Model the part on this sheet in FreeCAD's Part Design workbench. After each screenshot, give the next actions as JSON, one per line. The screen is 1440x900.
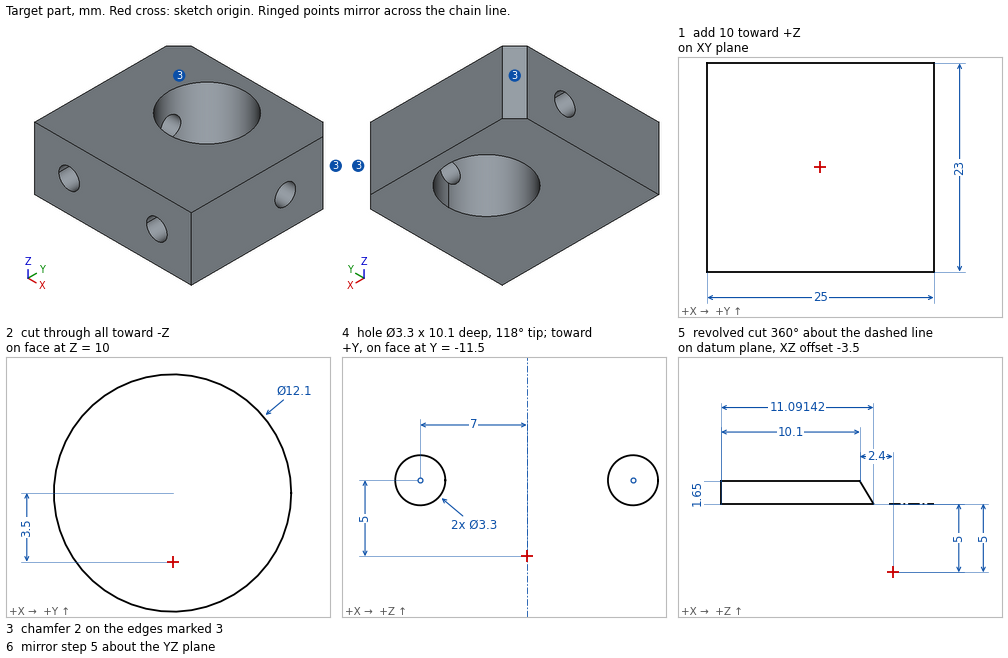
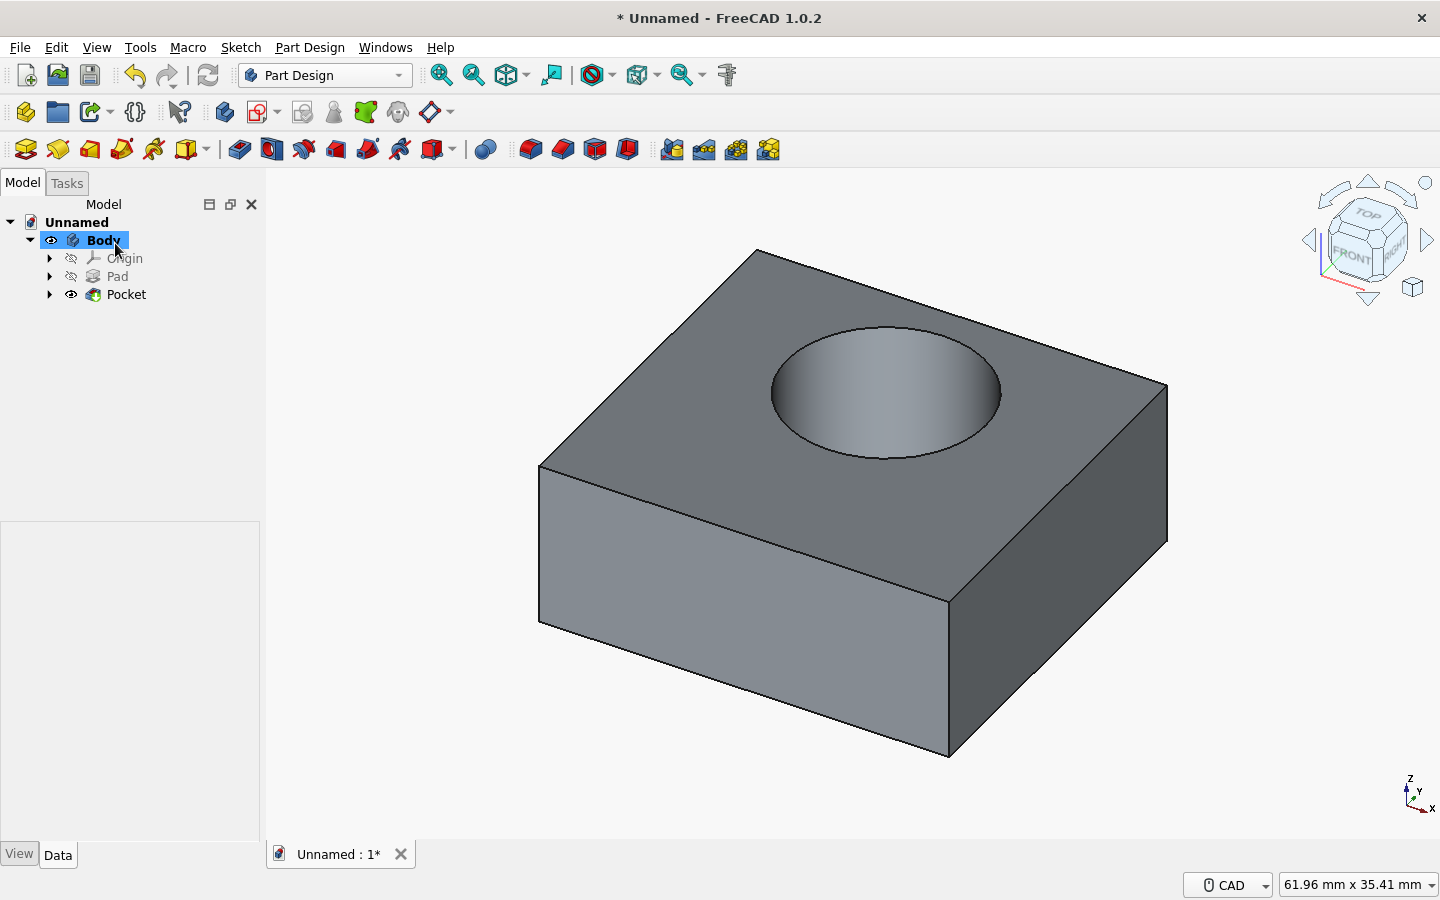
{"action": "key", "text": "0"}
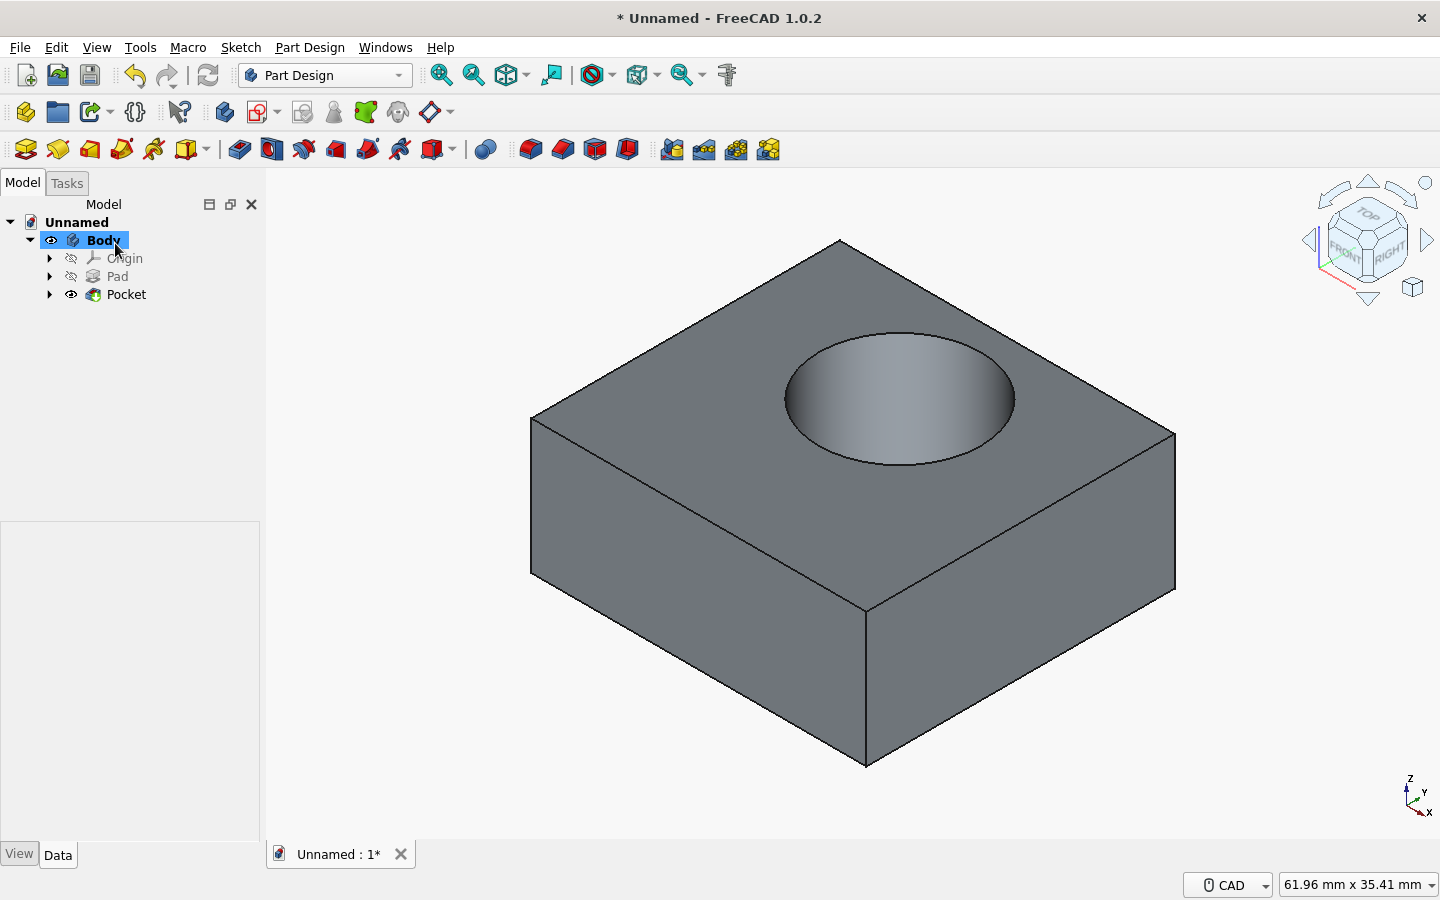
{"action": "key", "text": "2"}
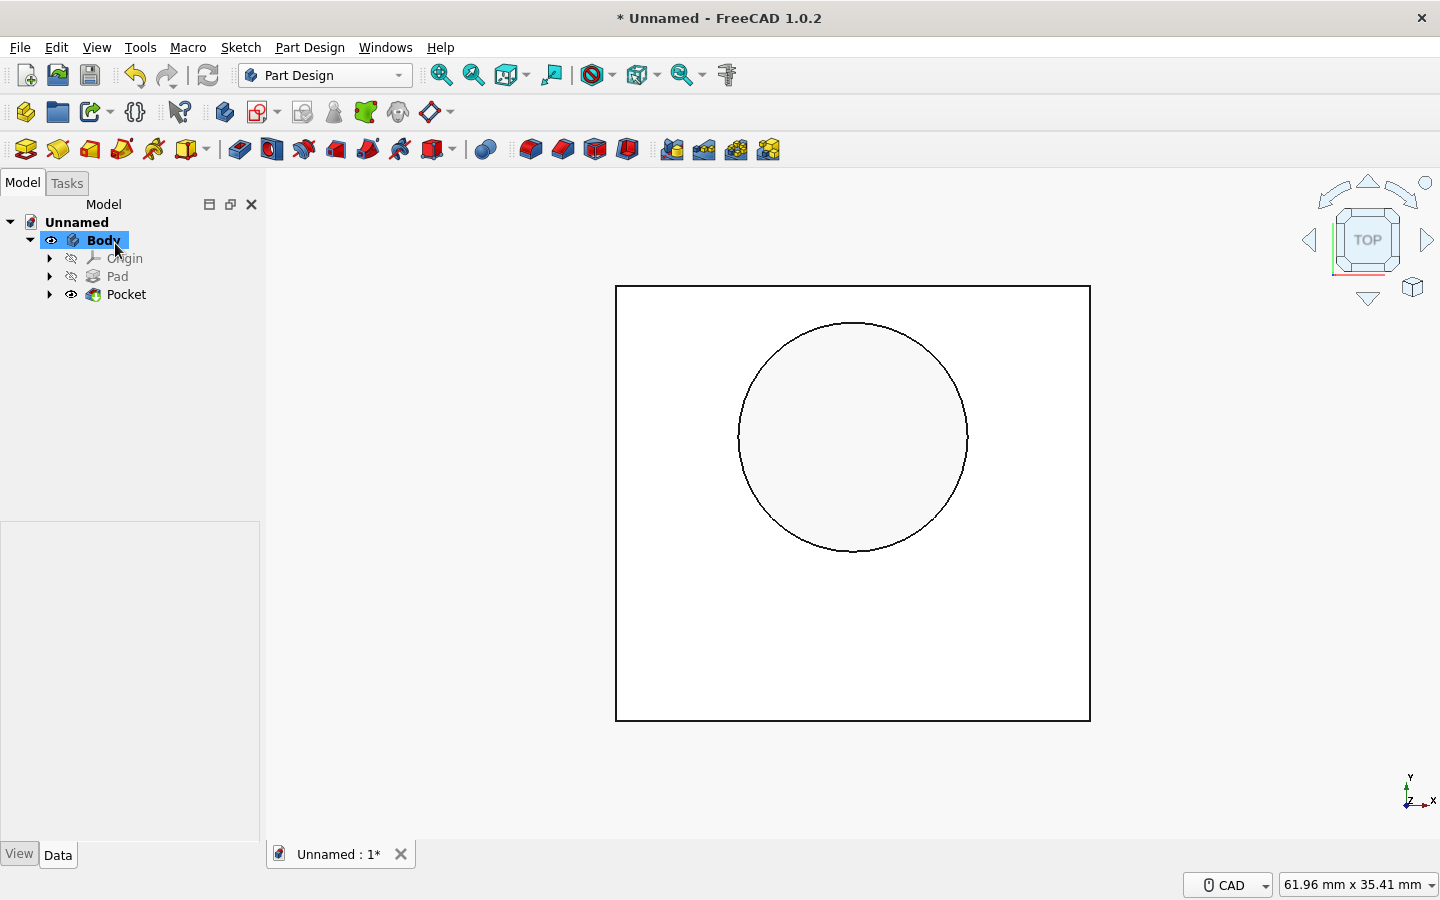
{"action": "key", "text": "1"}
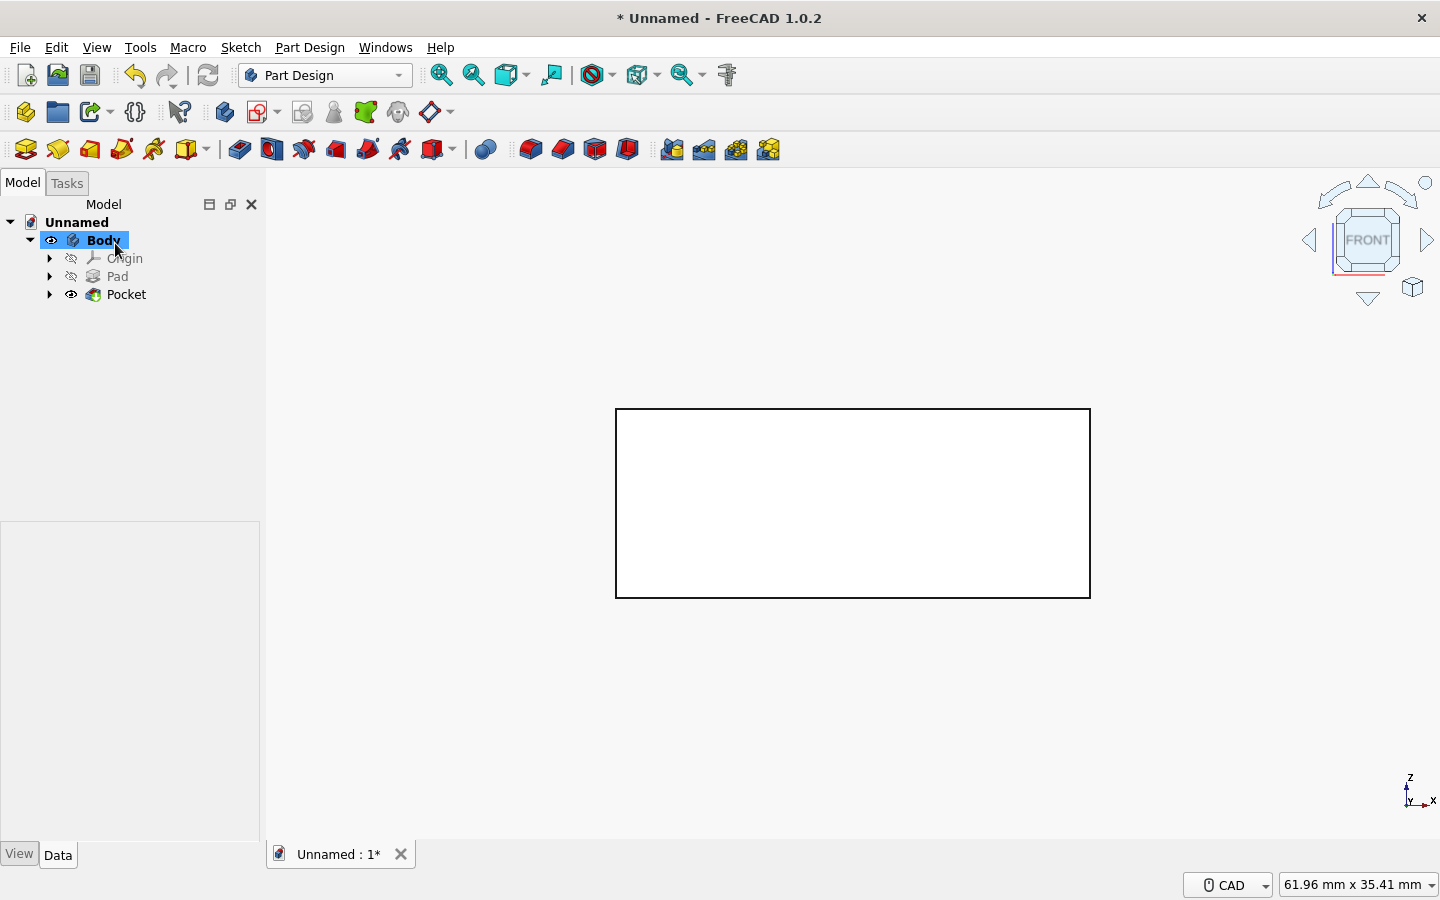
{"action": "left_click", "coordinate": [442, 76]}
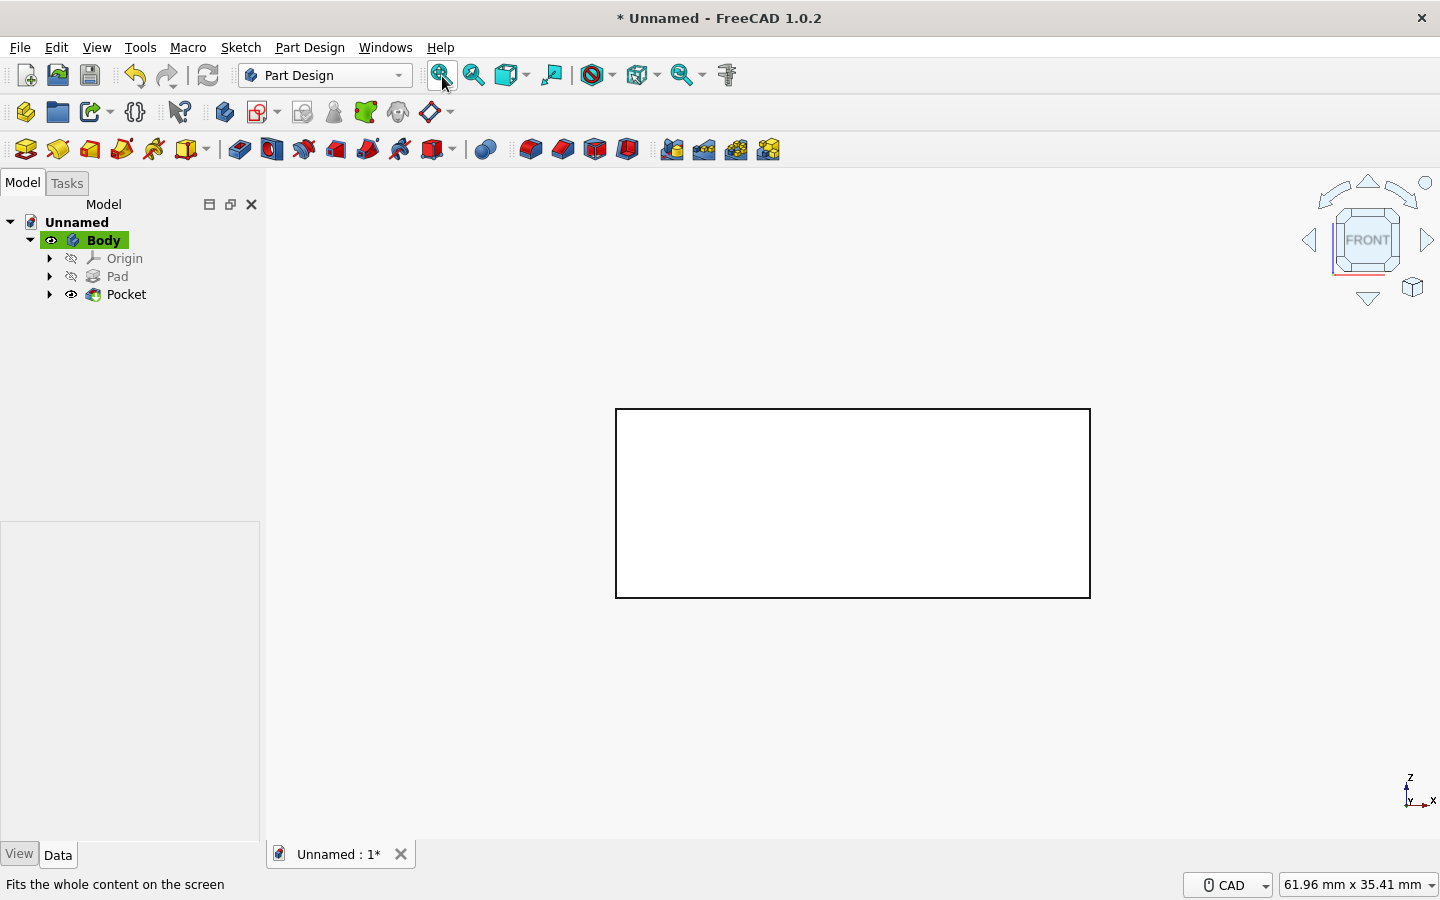
{"action": "key", "text": "3"}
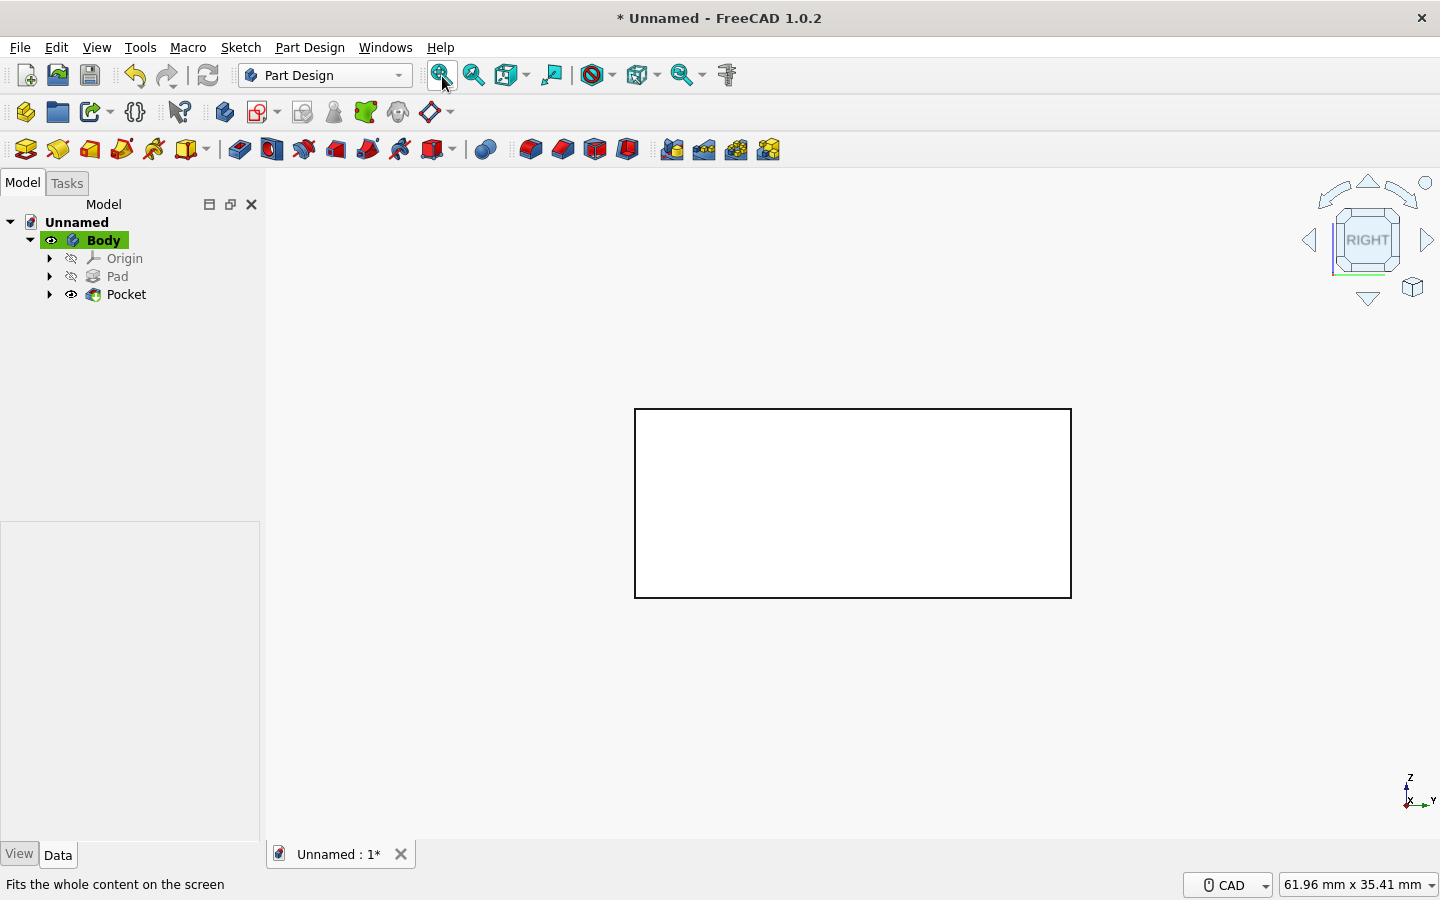
{"action": "key", "text": "v f"}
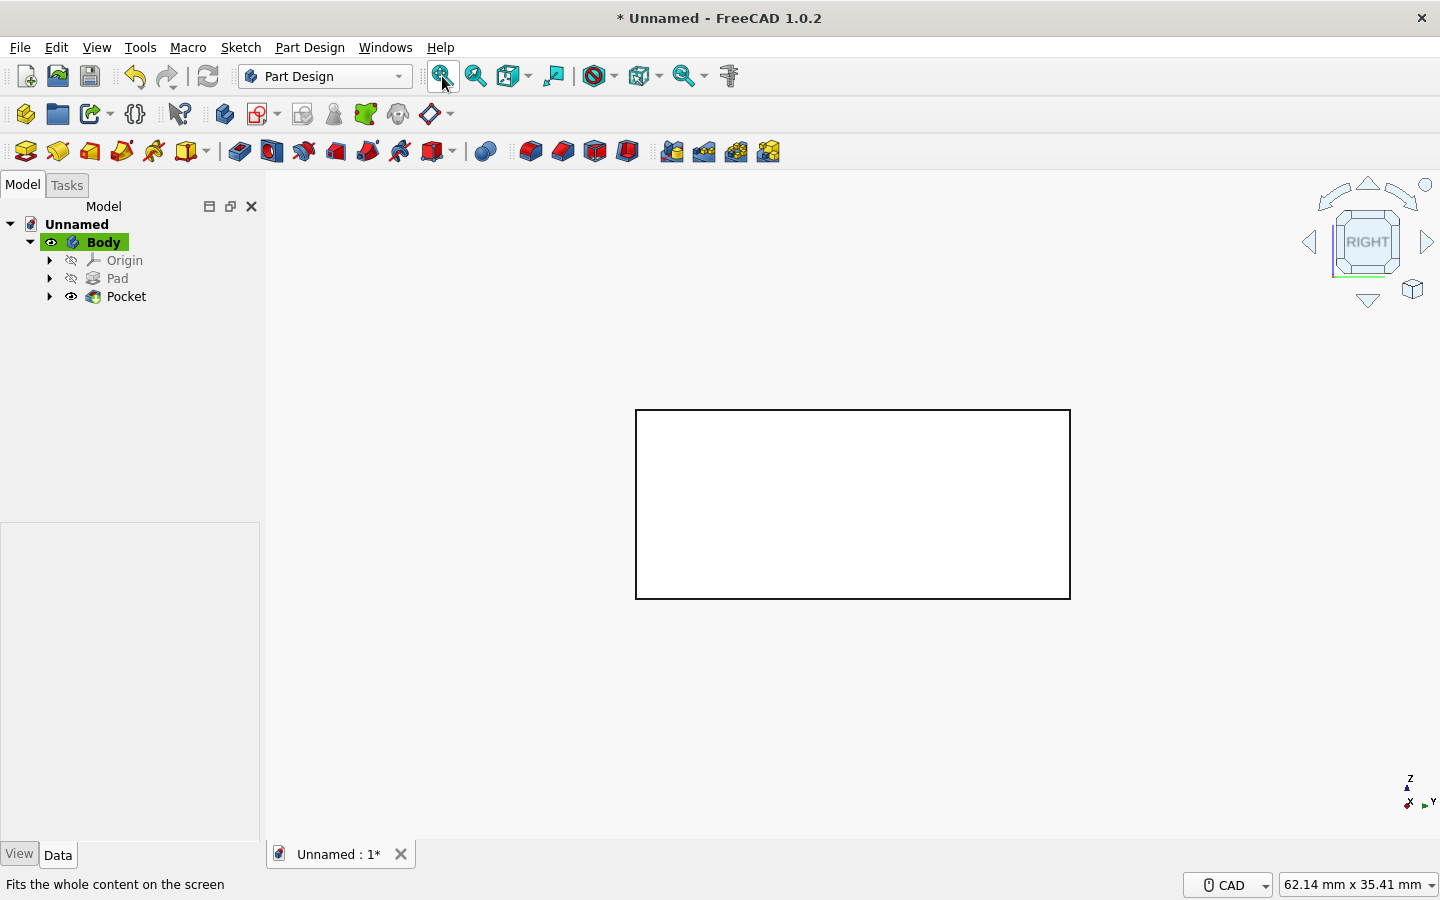
{"action": "left_click", "coordinate": [1070, 503]}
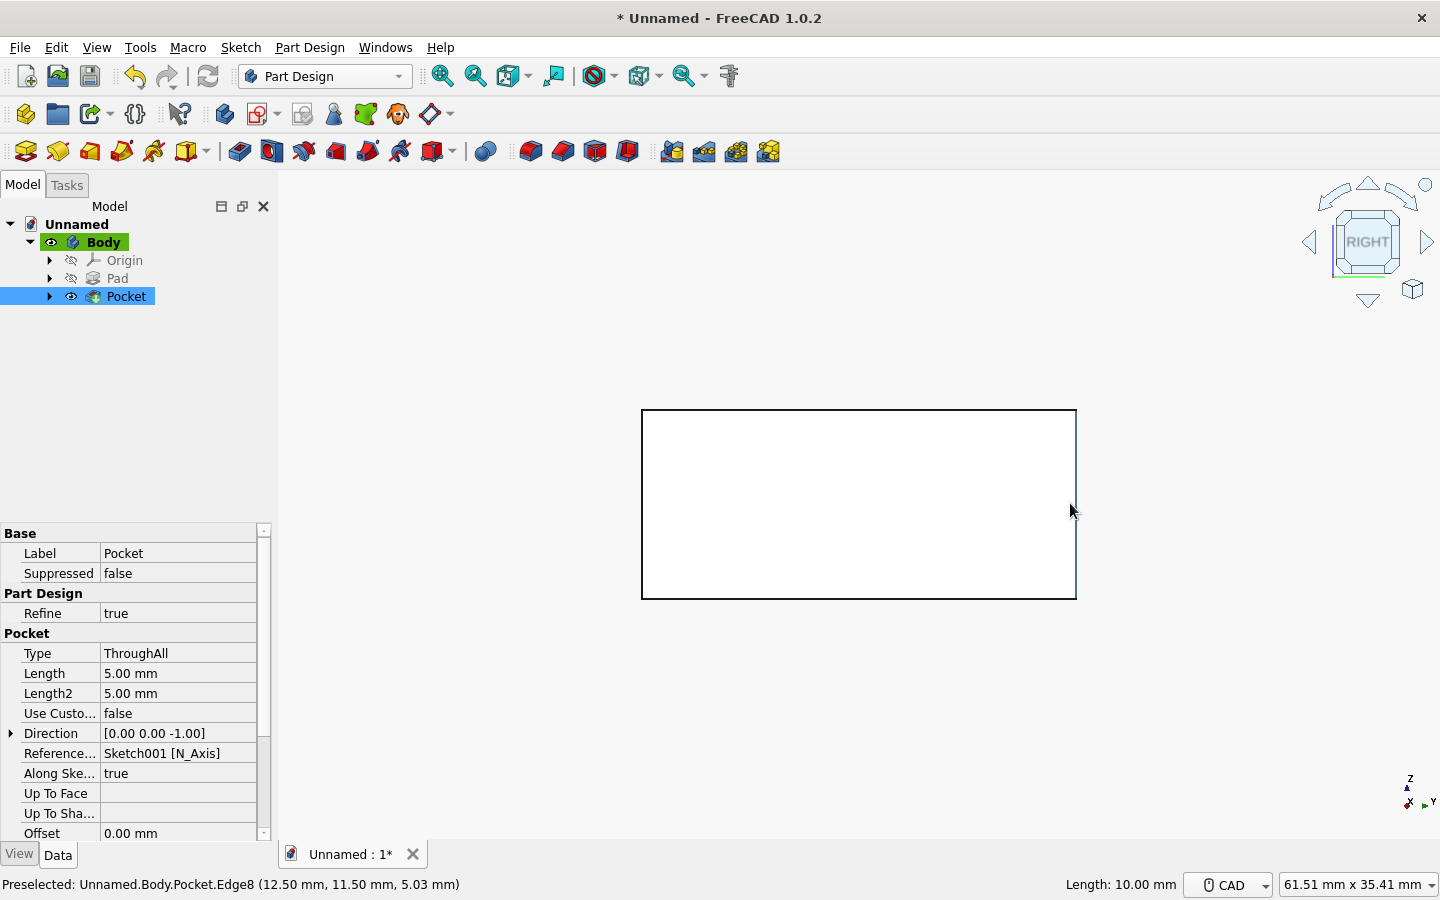
{"action": "key", "text": "5"}